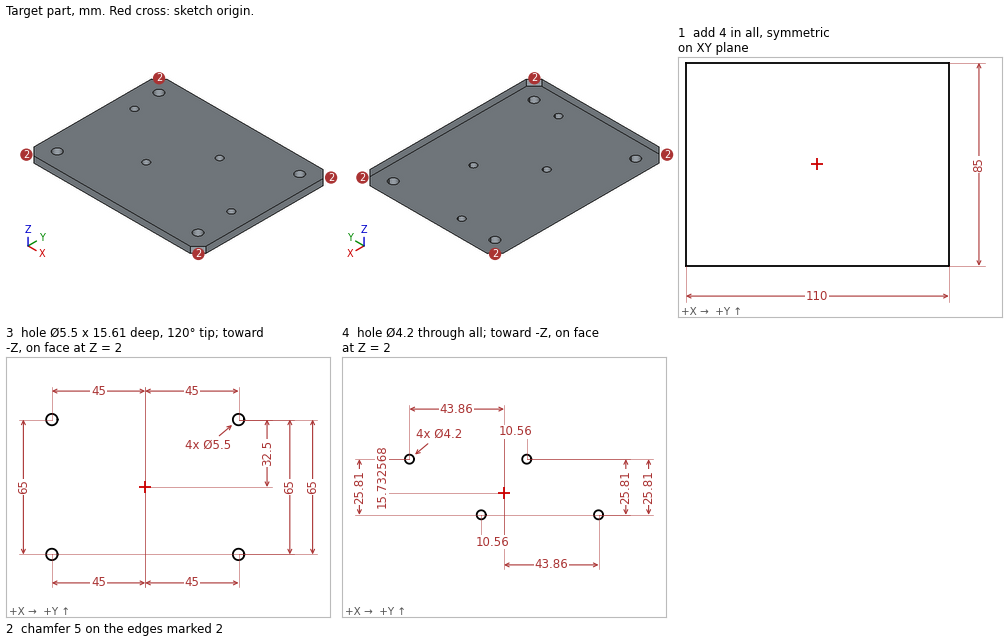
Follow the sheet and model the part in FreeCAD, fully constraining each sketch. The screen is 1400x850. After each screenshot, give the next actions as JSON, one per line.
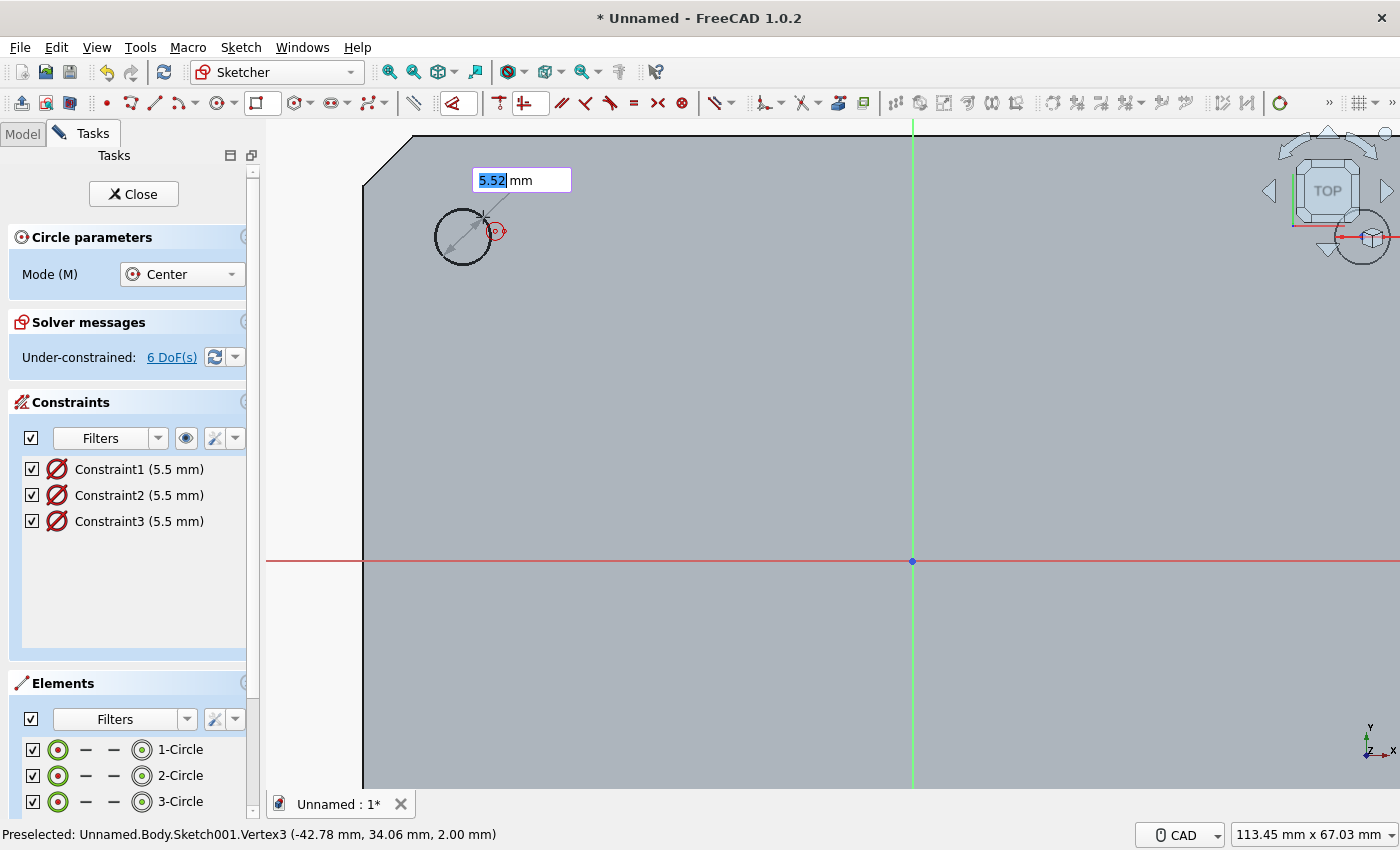
{"action": "type", "text": "5.5"}
{"action": "key", "text": "Return"}
{"action": "key", "text": "Escape"}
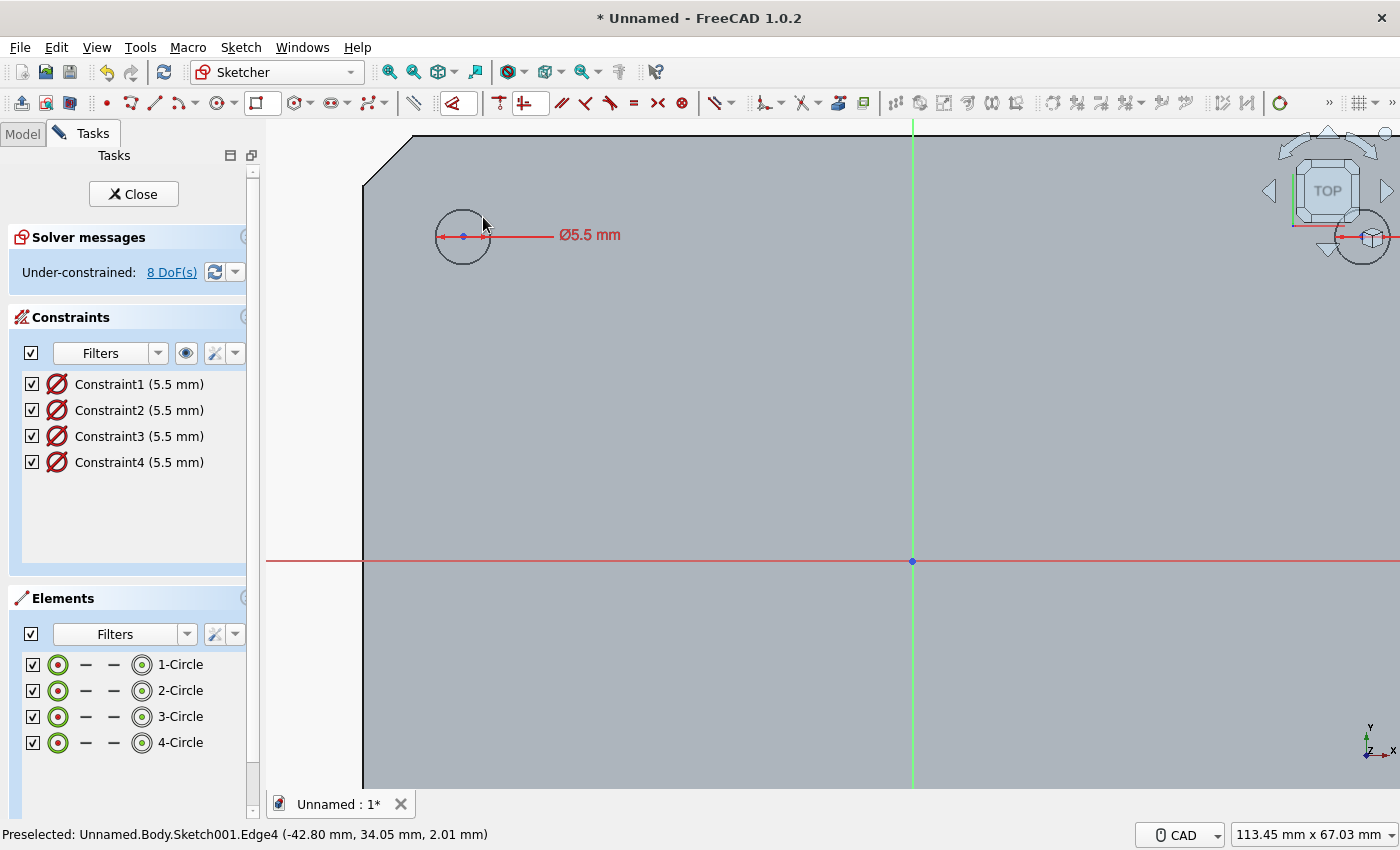
{"action": "left_click", "coordinate": [452, 104]}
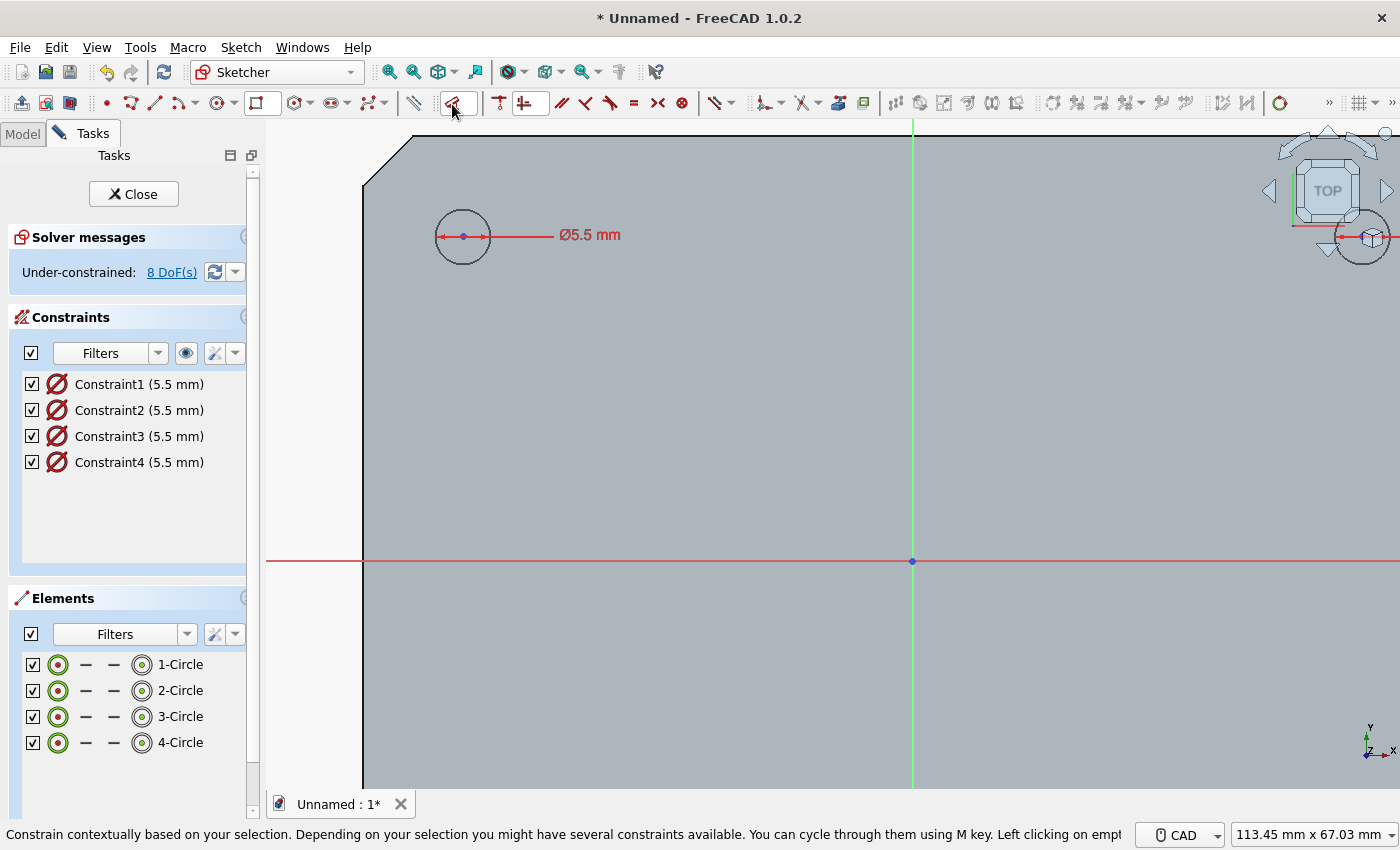
{"action": "scroll", "coordinate": [463, 236], "scroll_direction": "down", "scroll_amount": 2}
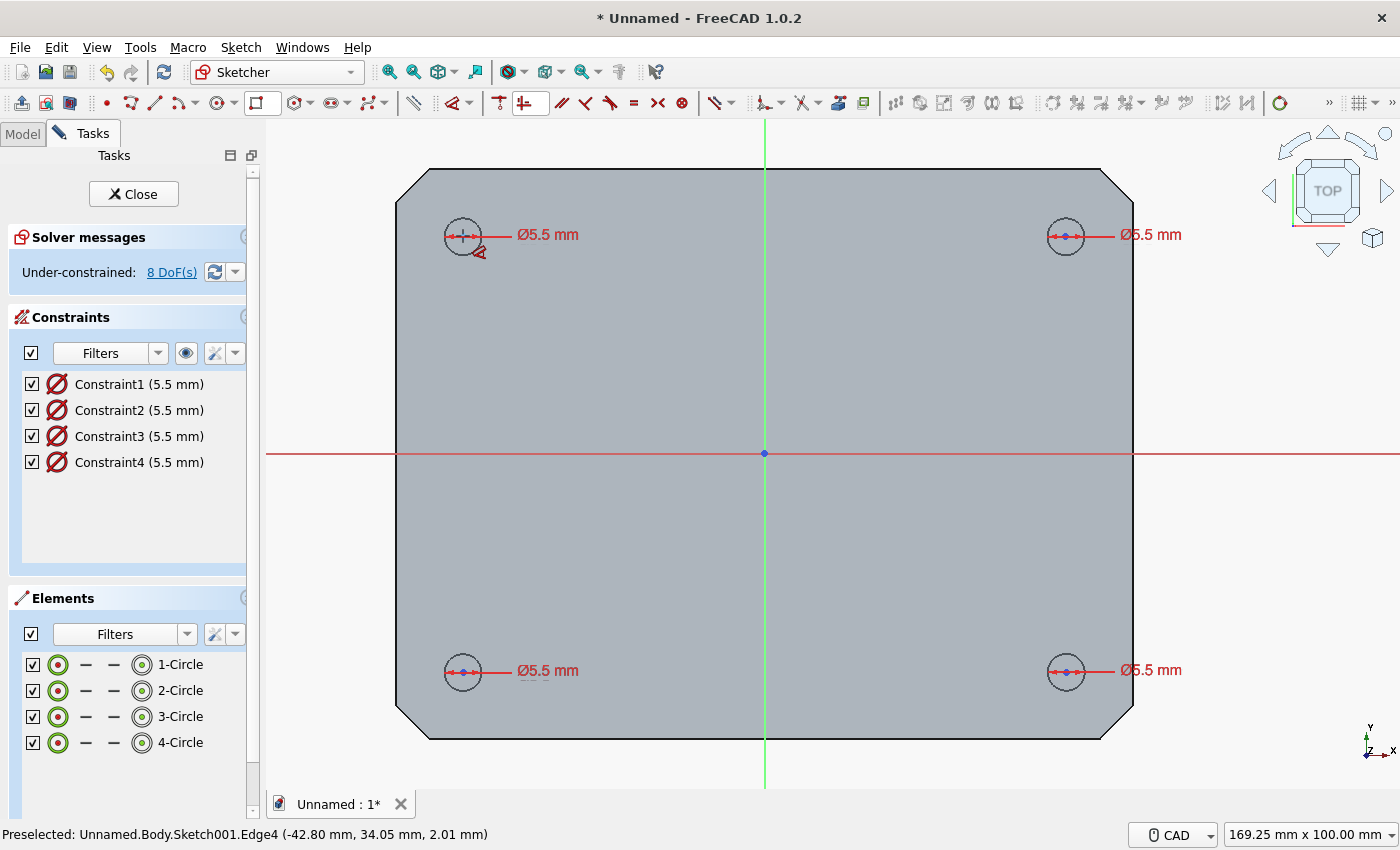
{"action": "left_click", "coordinate": [1066, 237]}
{"action": "left_click", "coordinate": [915, 203]}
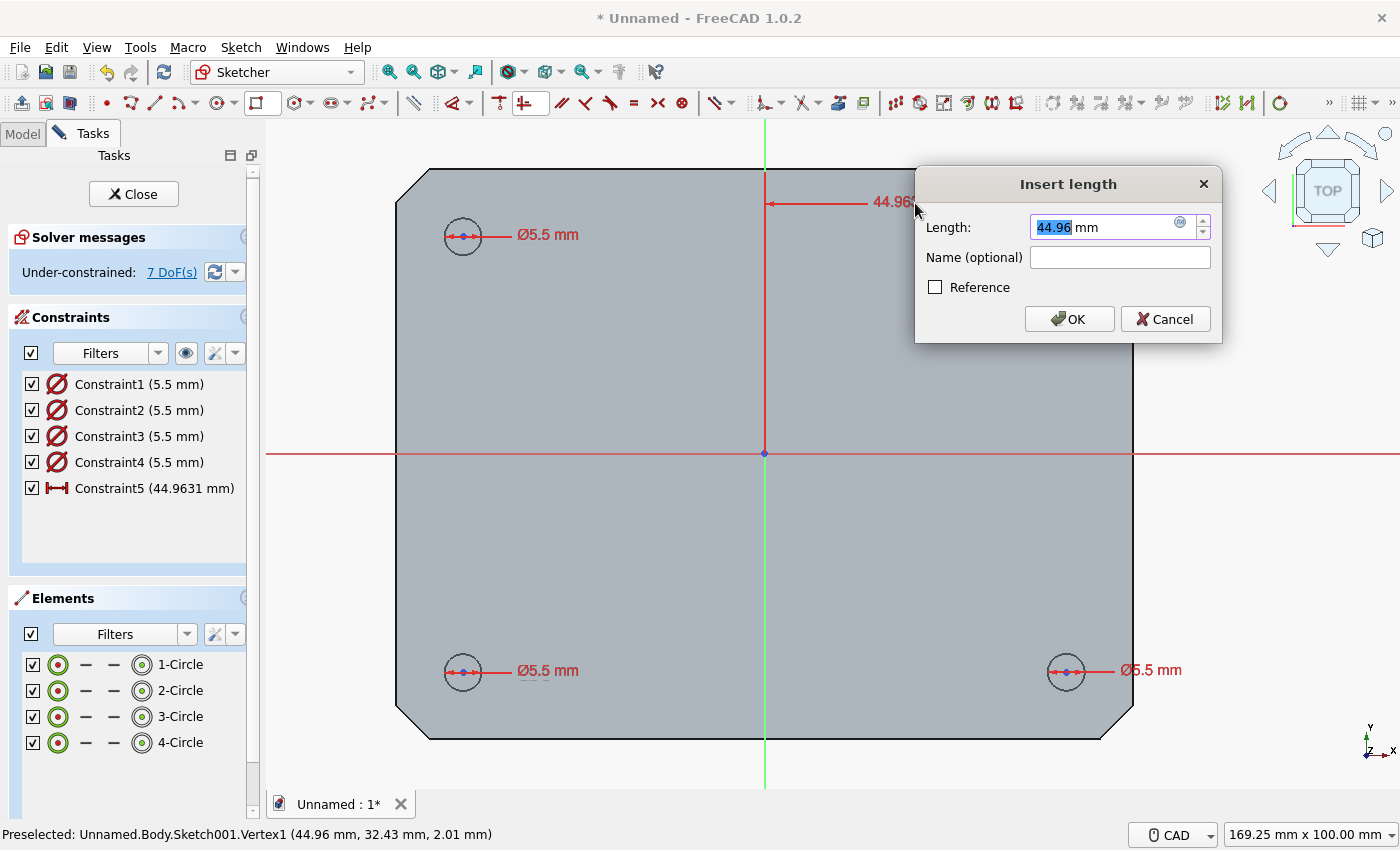
{"action": "type", "text": "45"}
{"action": "key", "text": "Return"}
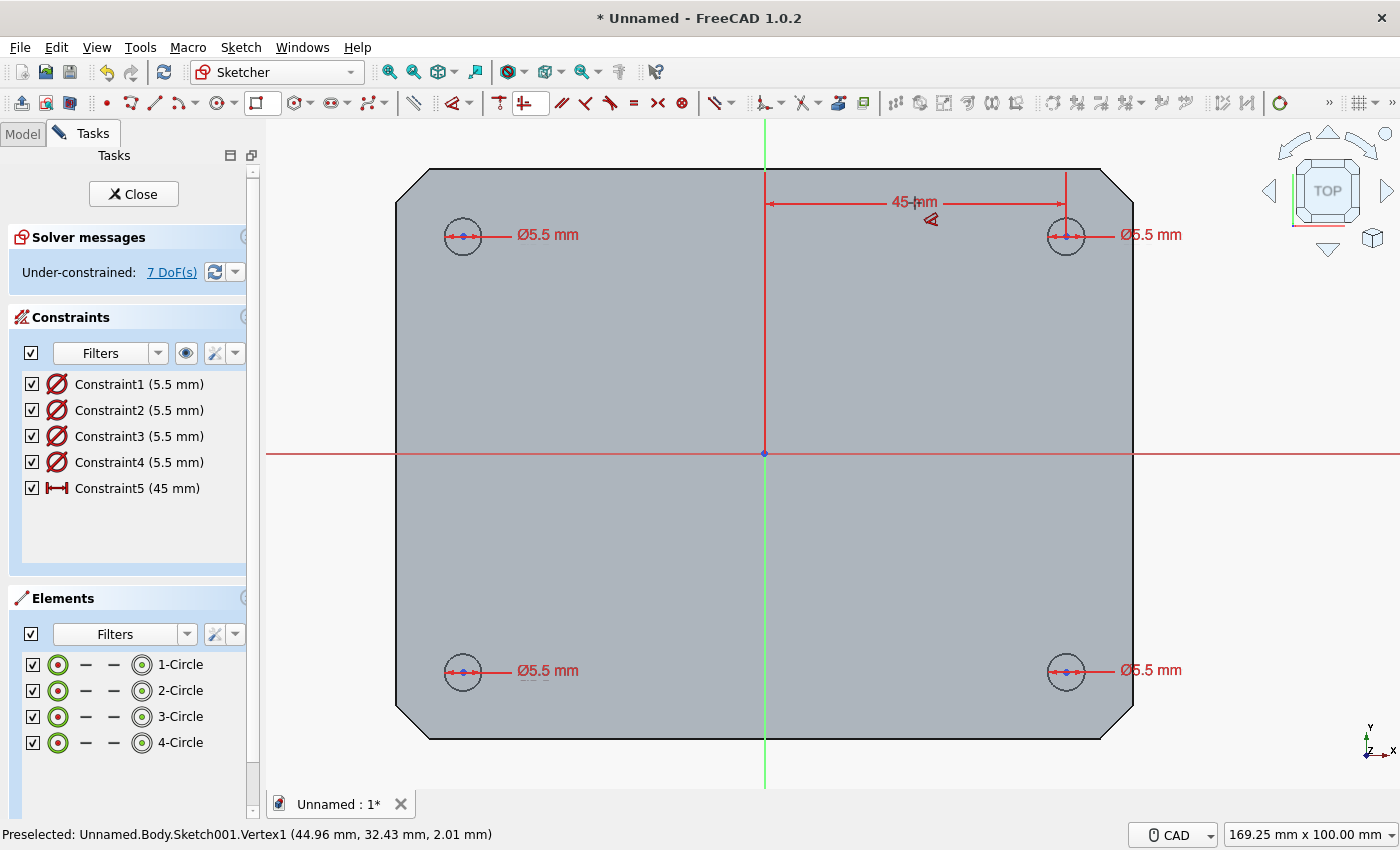
{"action": "left_click", "coordinate": [1066, 672]}
{"action": "left_click", "coordinate": [915, 706]}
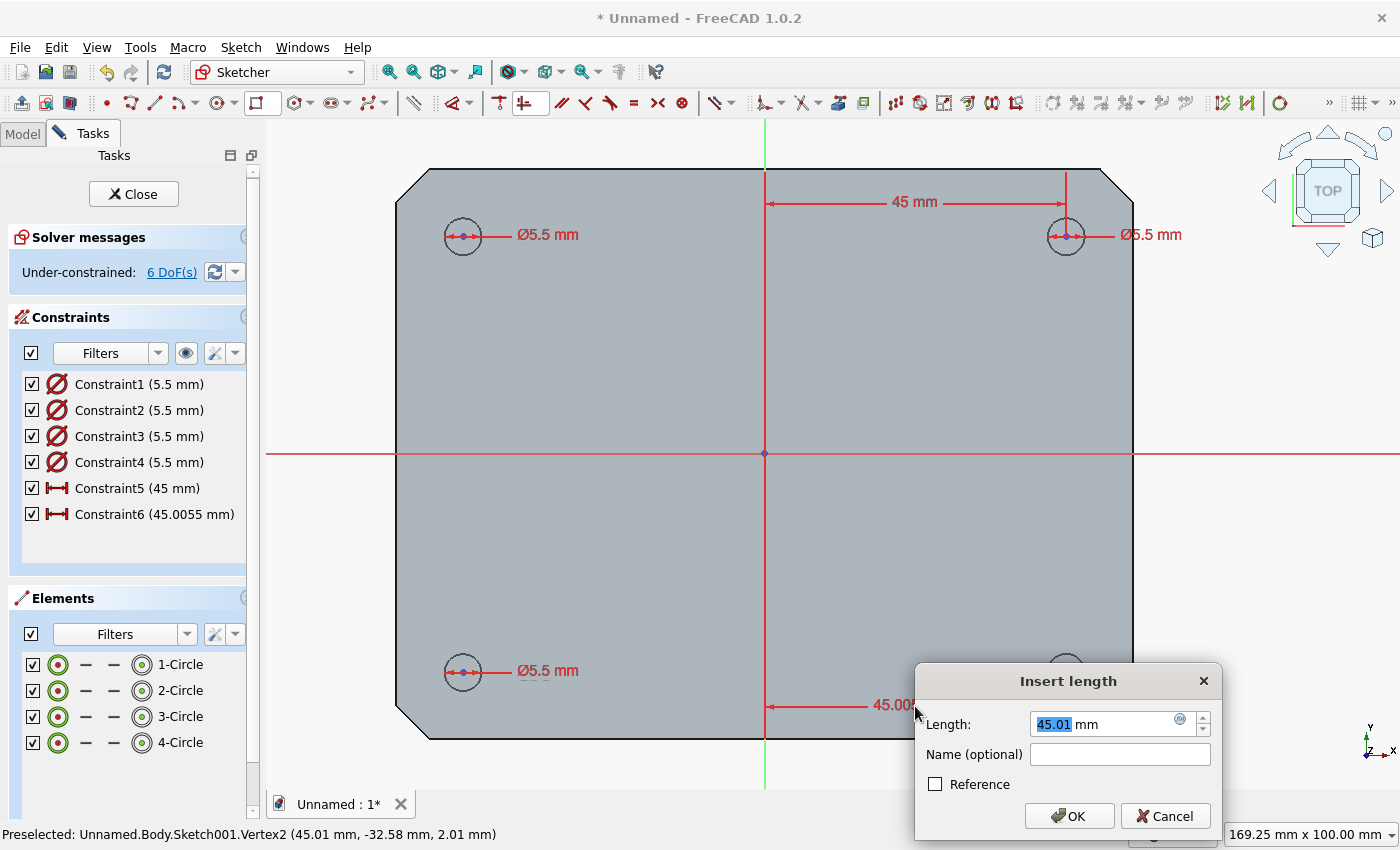
{"action": "type", "text": "45"}
{"action": "key", "text": "Return"}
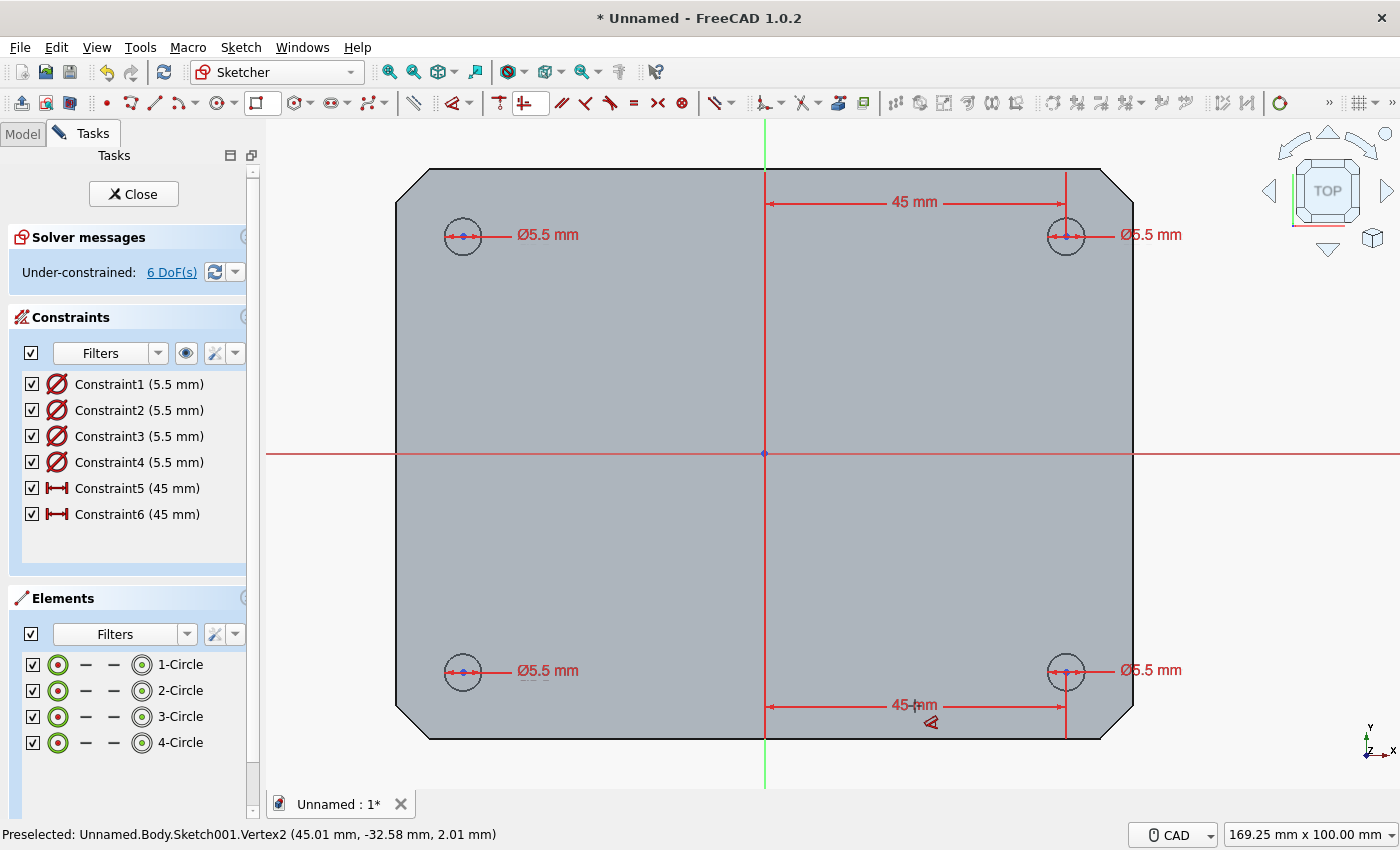
{"action": "left_click", "coordinate": [463, 673]}
{"action": "left_click", "coordinate": [614, 707]}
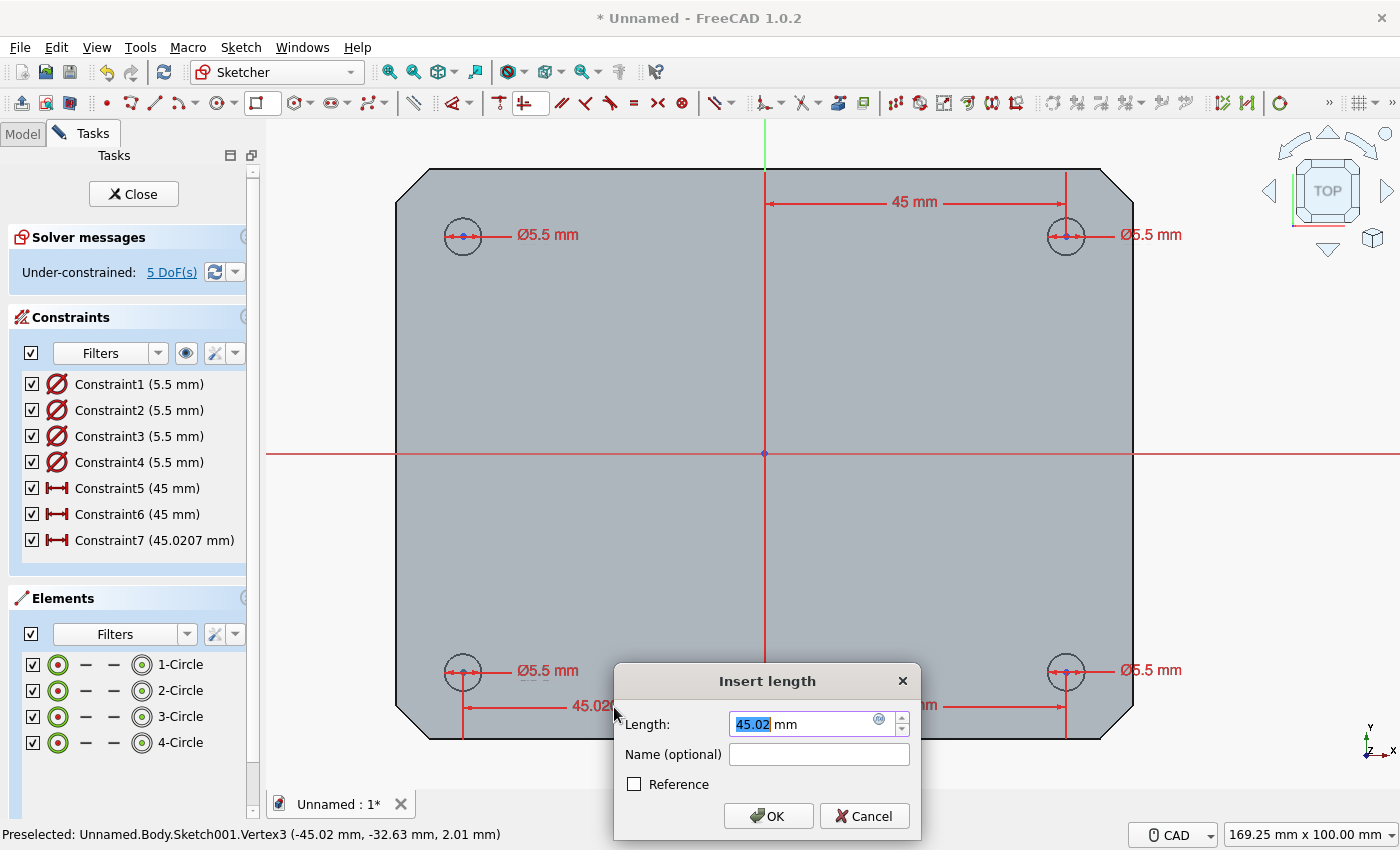
{"action": "type", "text": "45"}
{"action": "key", "text": "Return"}